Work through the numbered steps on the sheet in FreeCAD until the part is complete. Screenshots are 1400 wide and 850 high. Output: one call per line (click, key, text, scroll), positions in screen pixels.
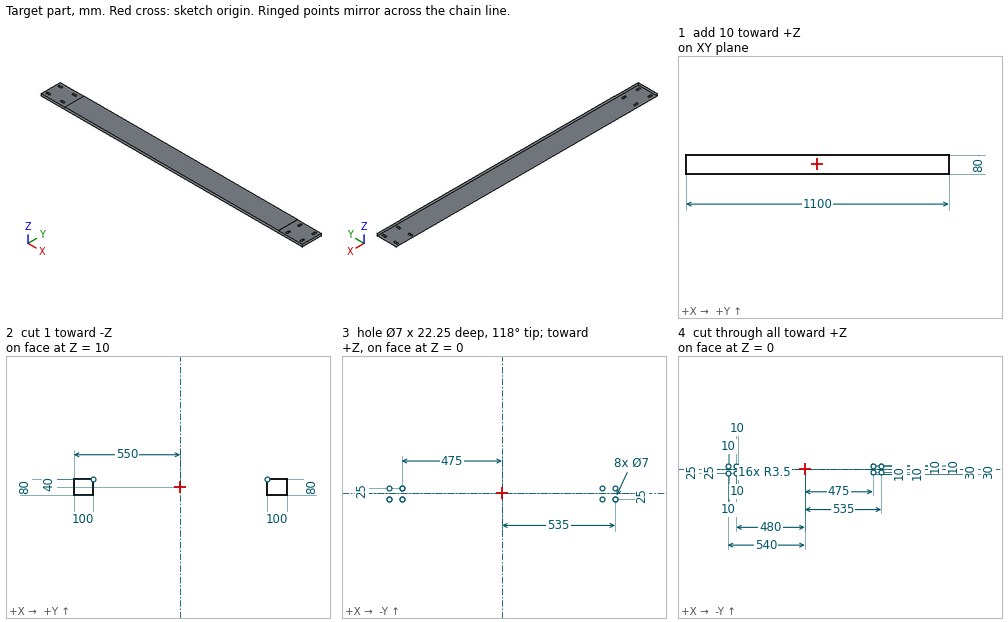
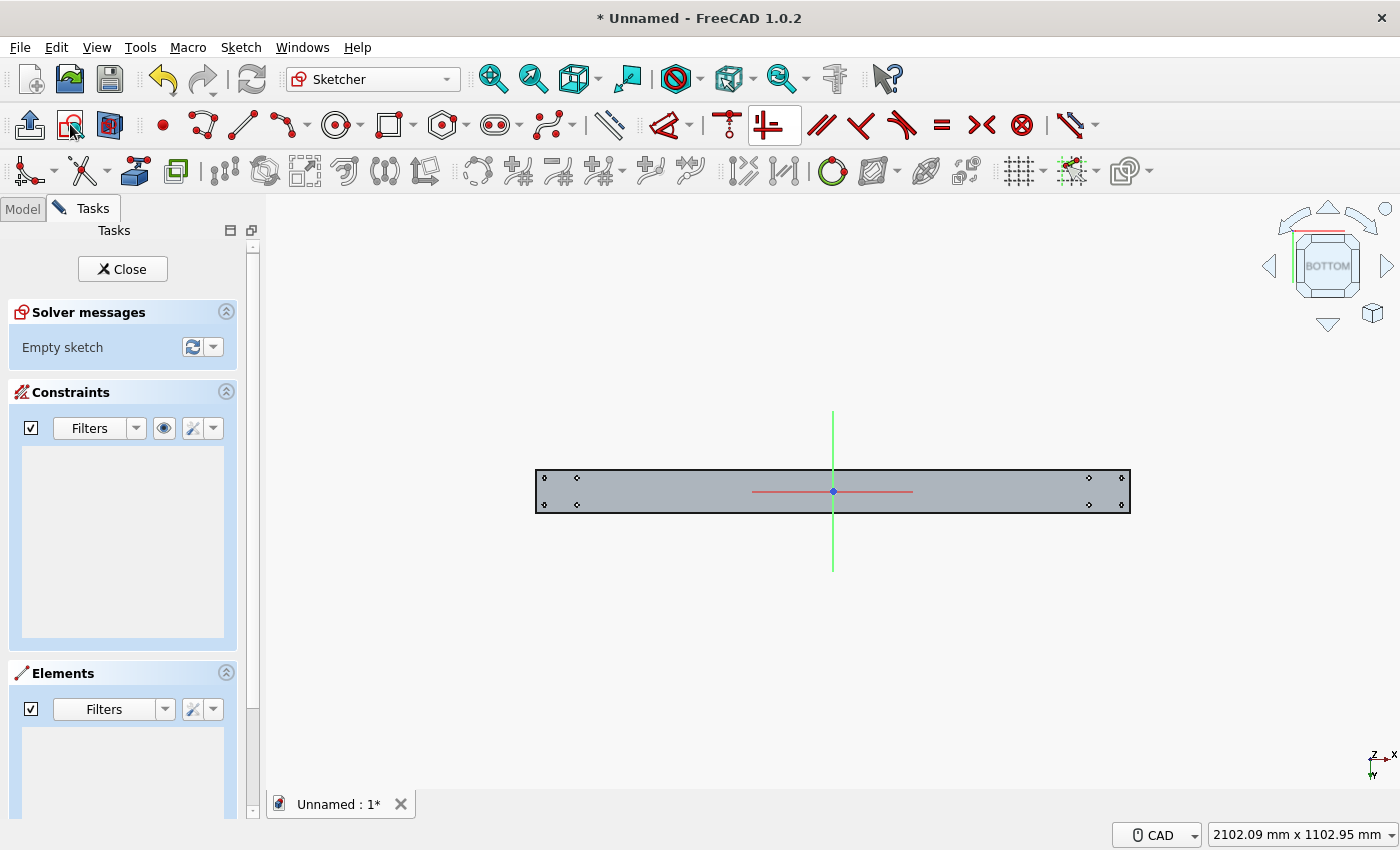
scroll(574, 505, up, 13)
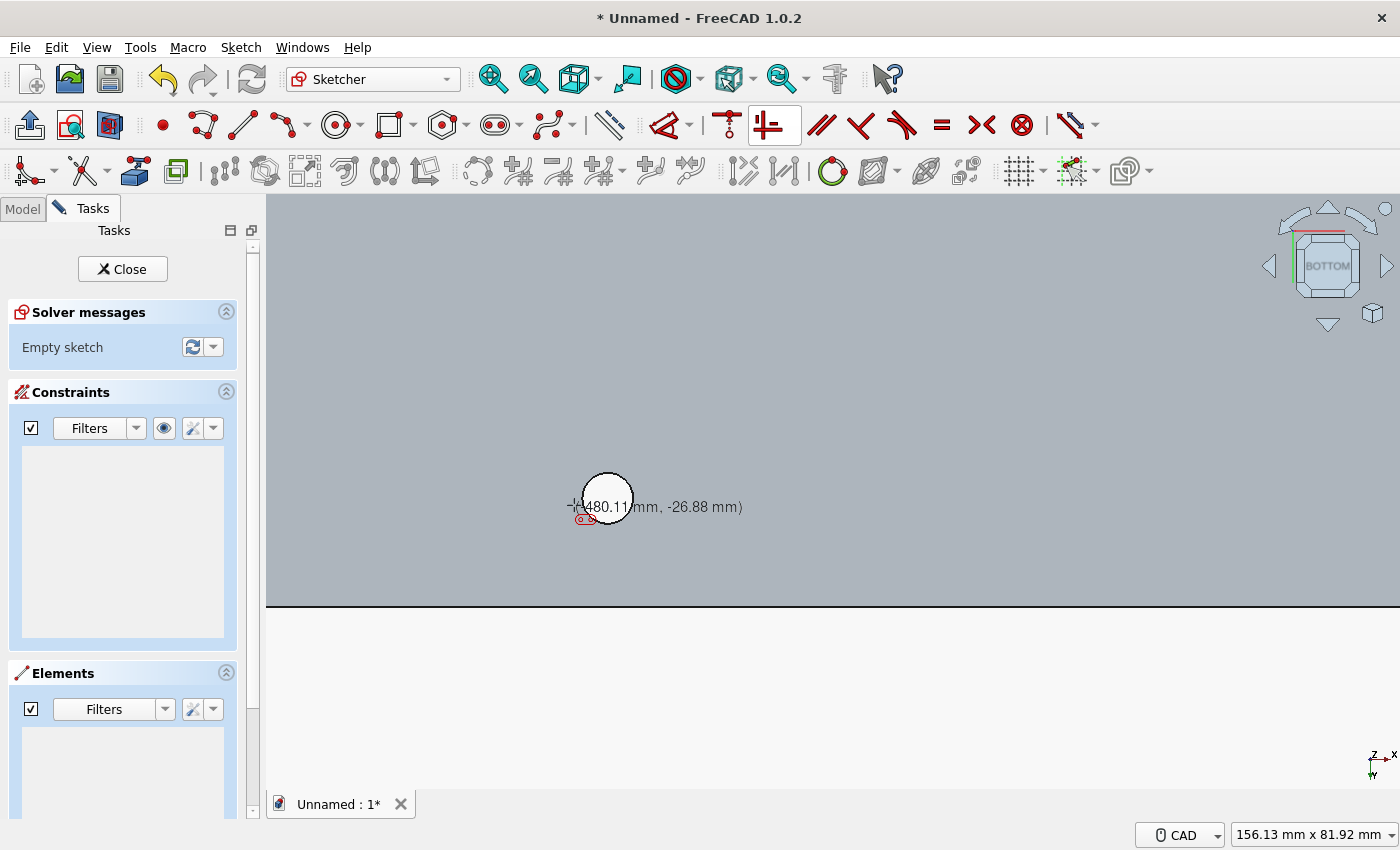
scroll(438, 509, down, 12)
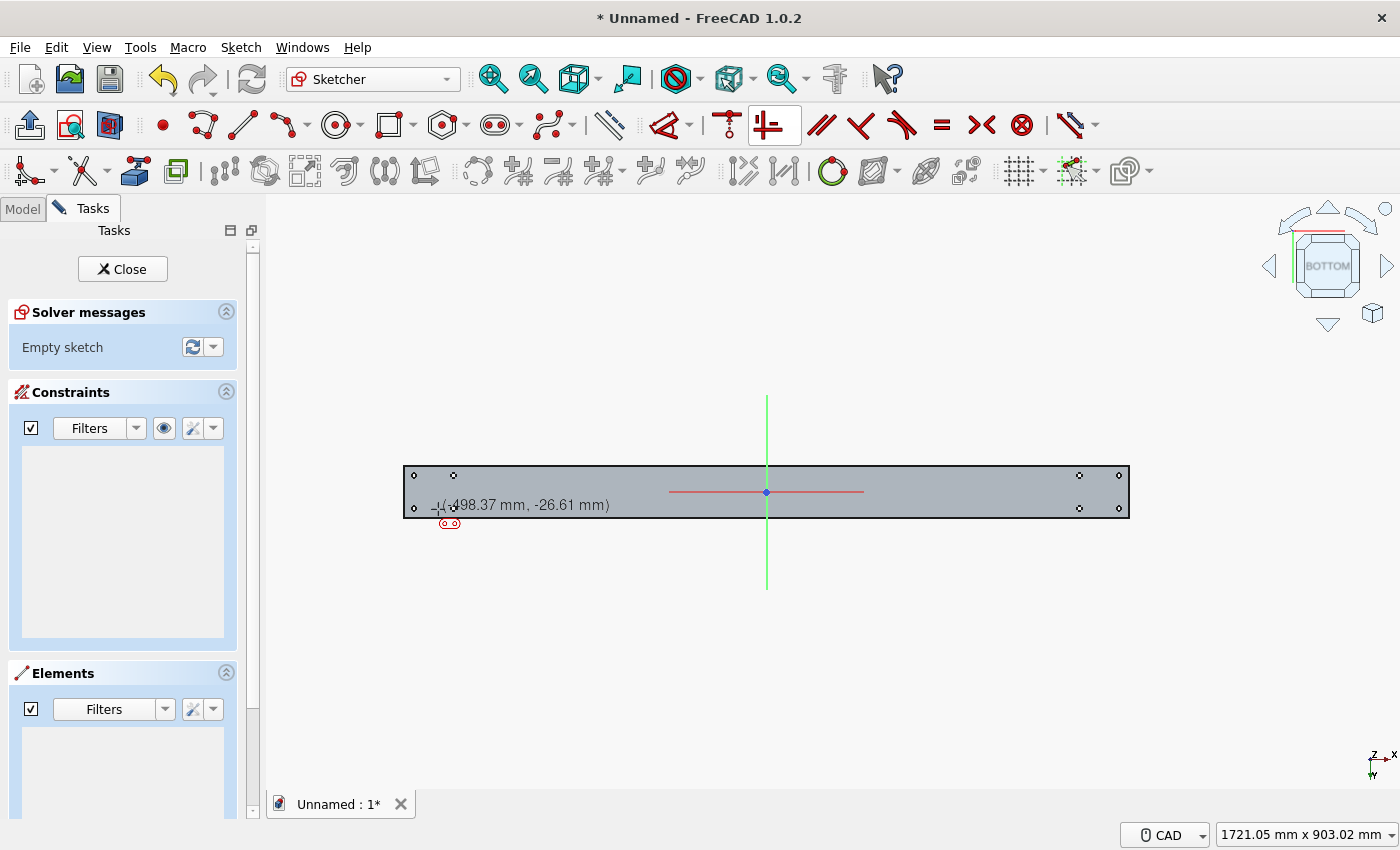
click(450, 509)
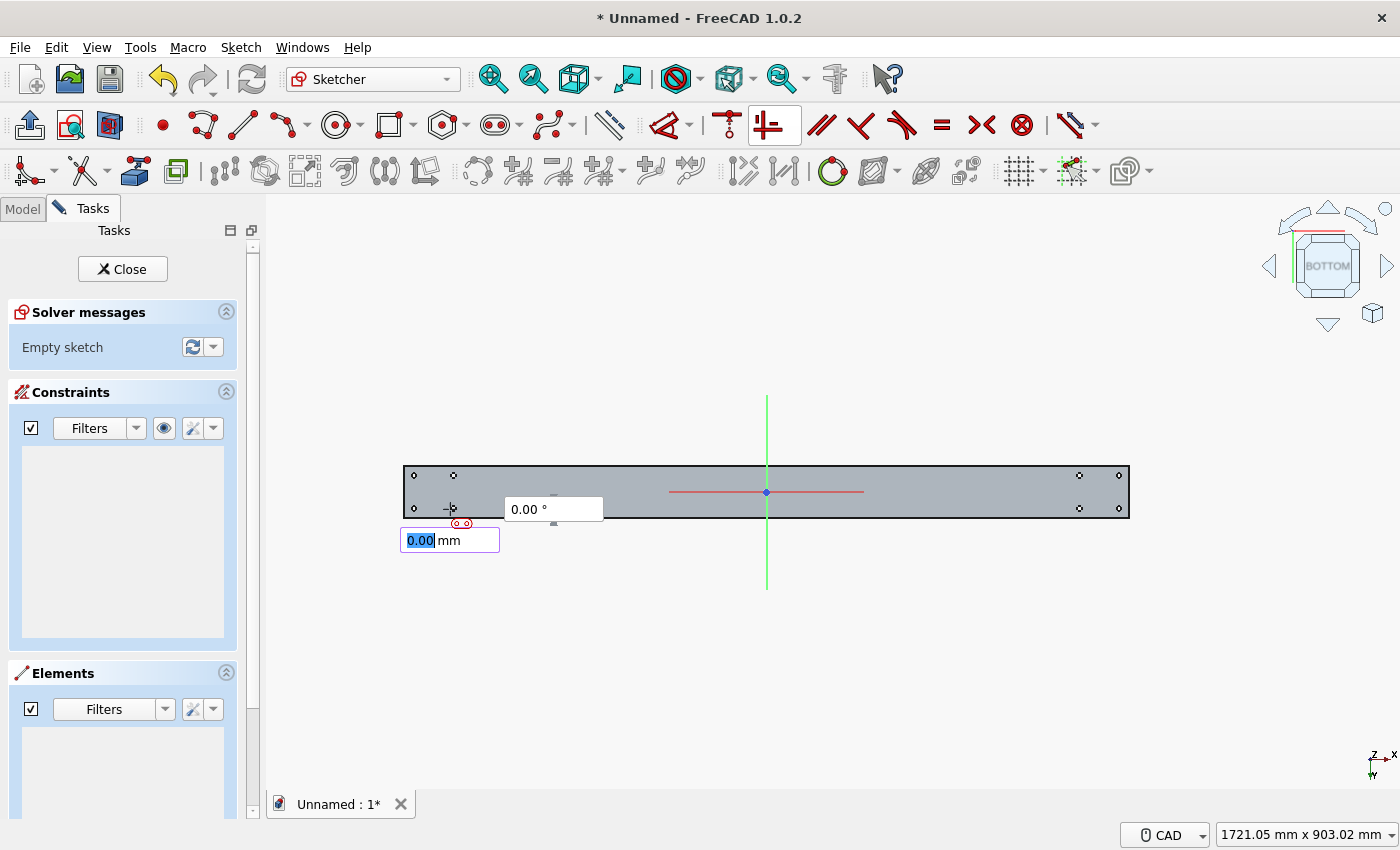
scroll(457, 509, up, 5)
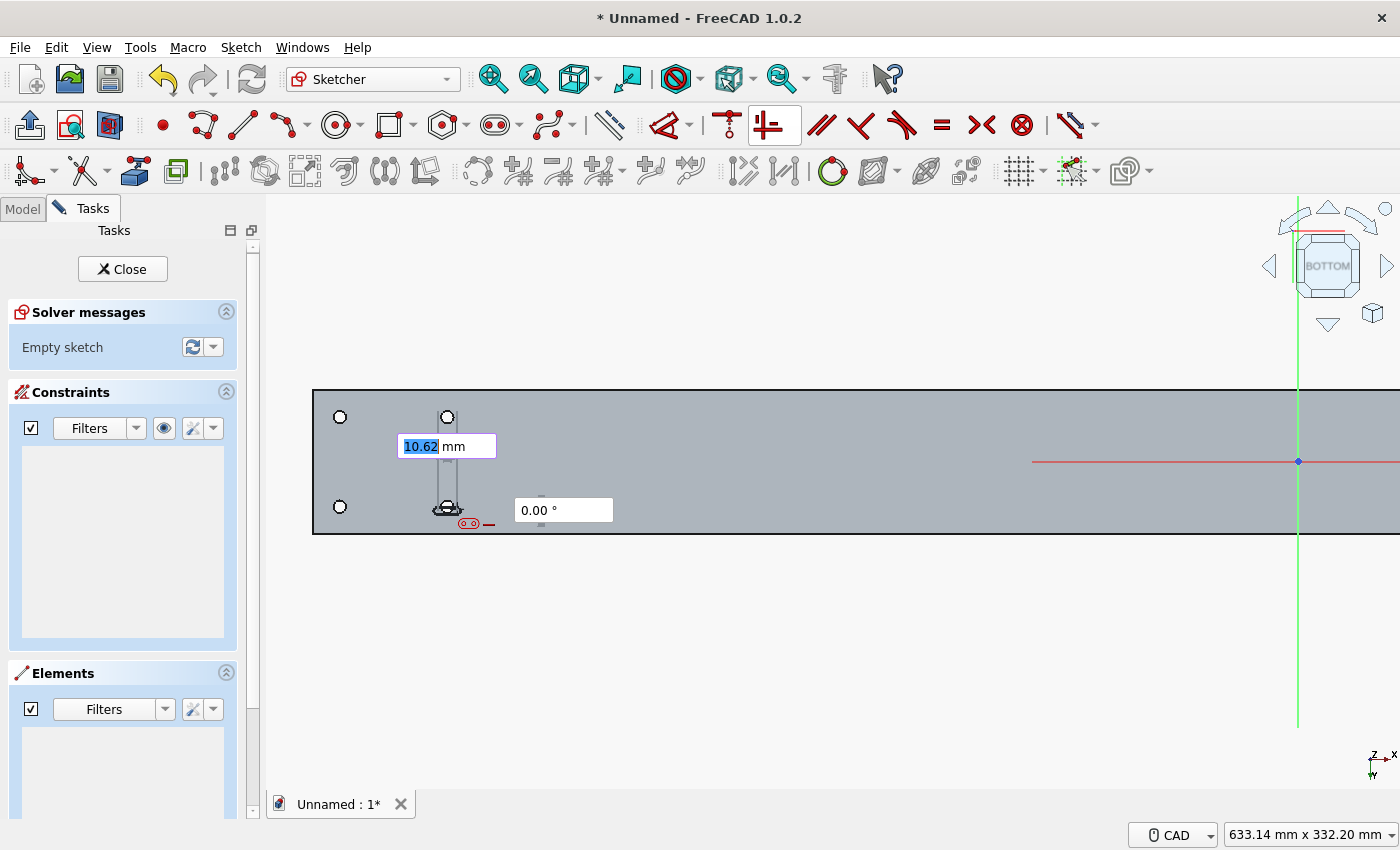
click(456, 508)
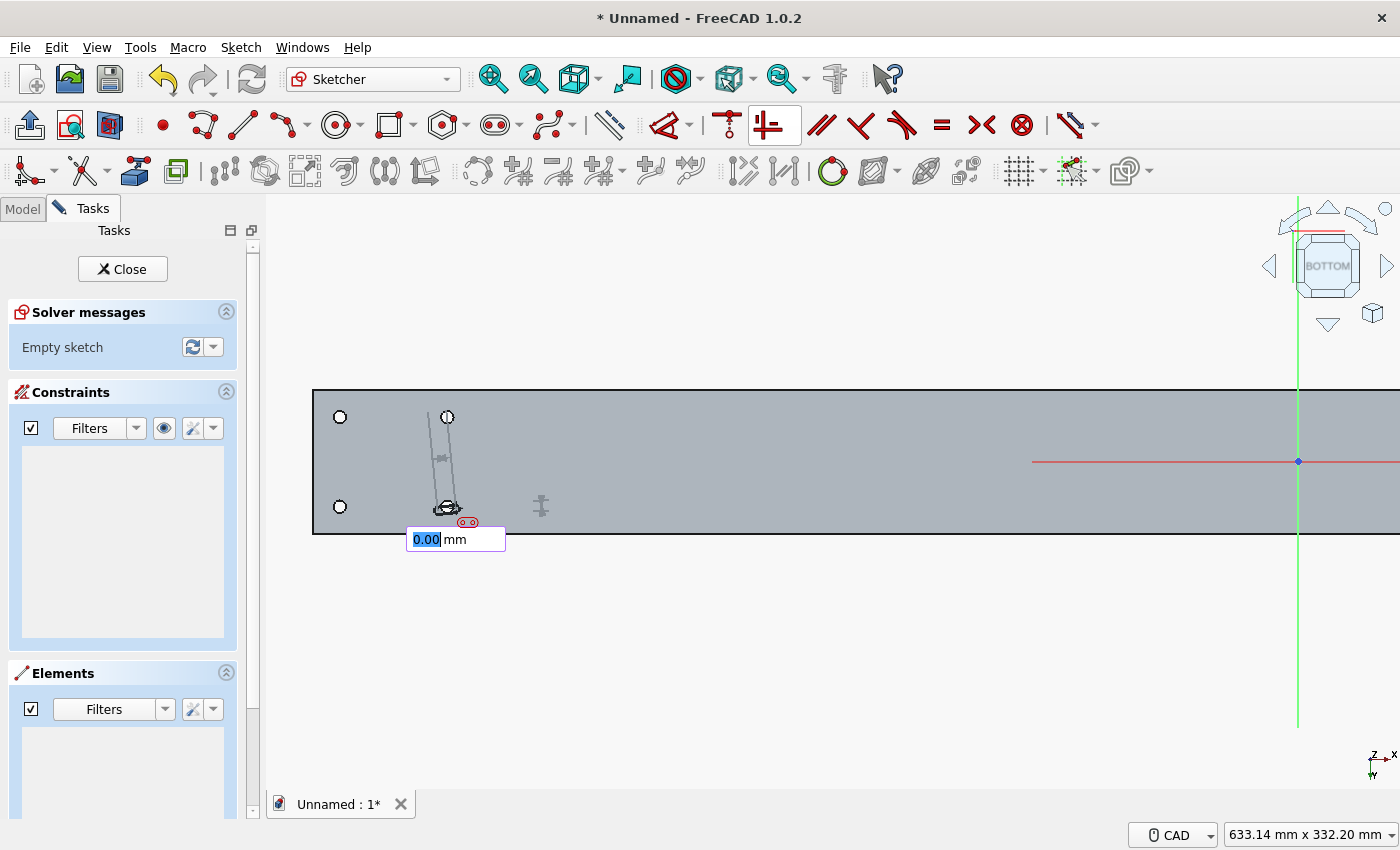
scroll(447, 513, up, 5)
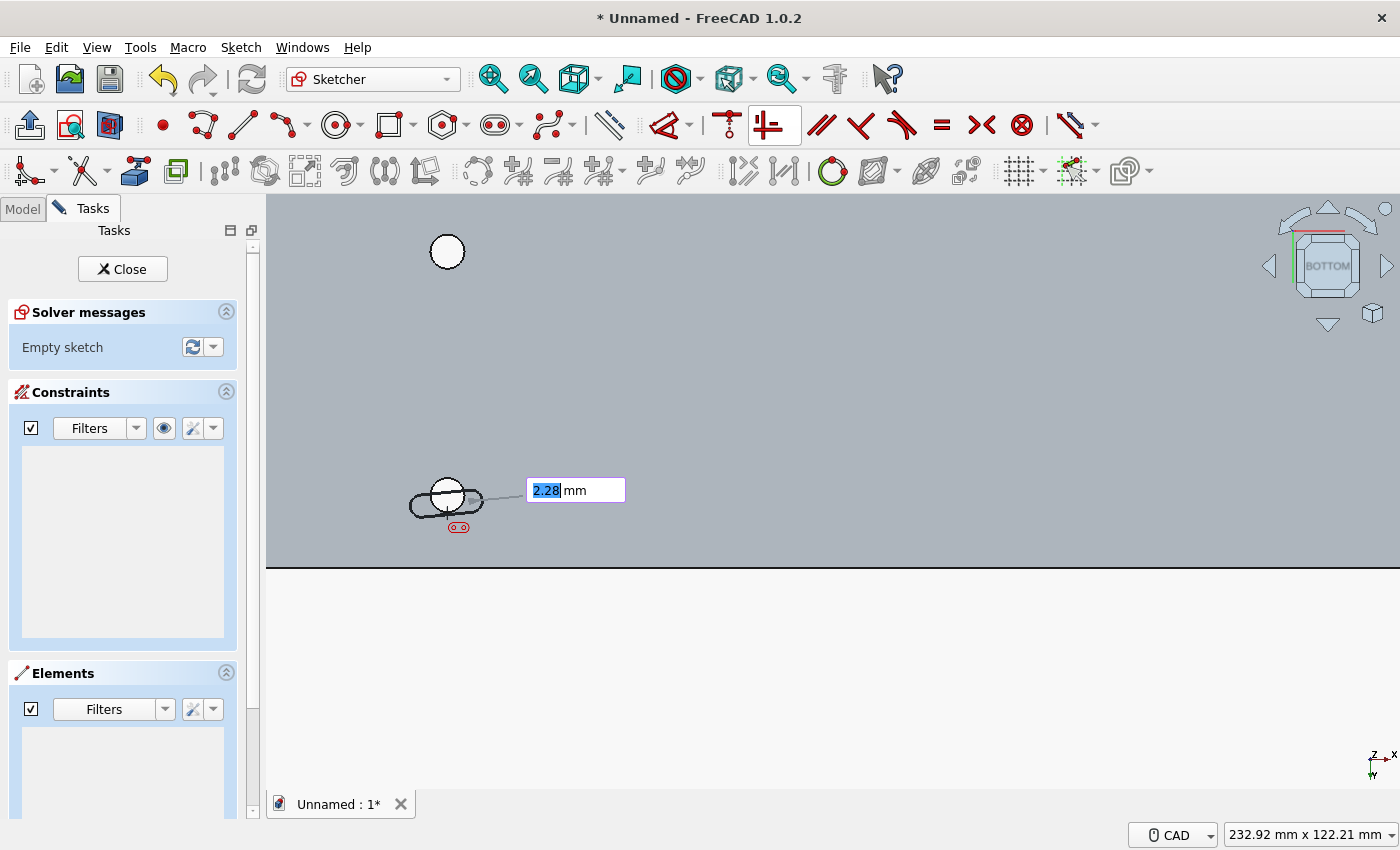
click(448, 512)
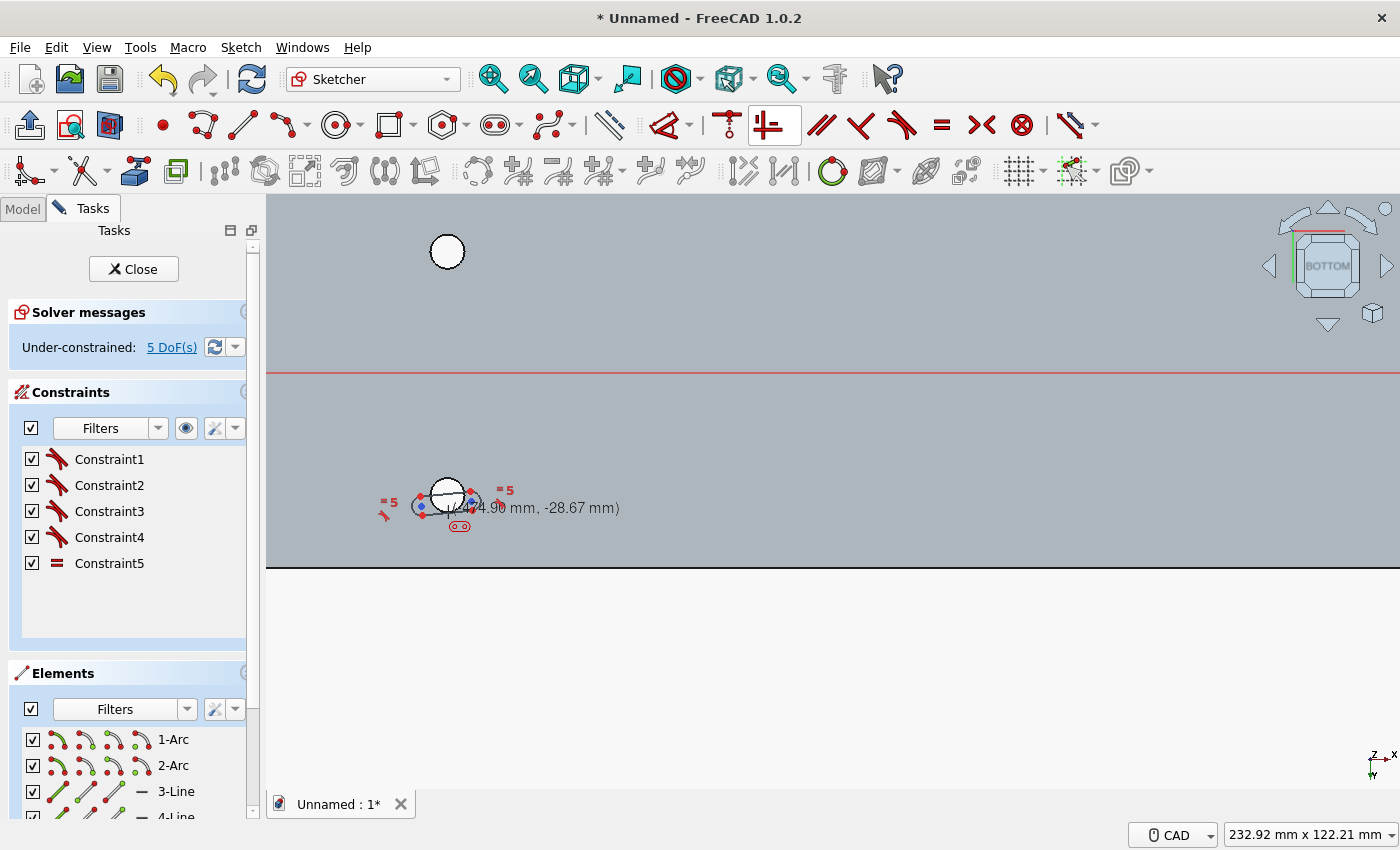
scroll(454, 510, down, 10)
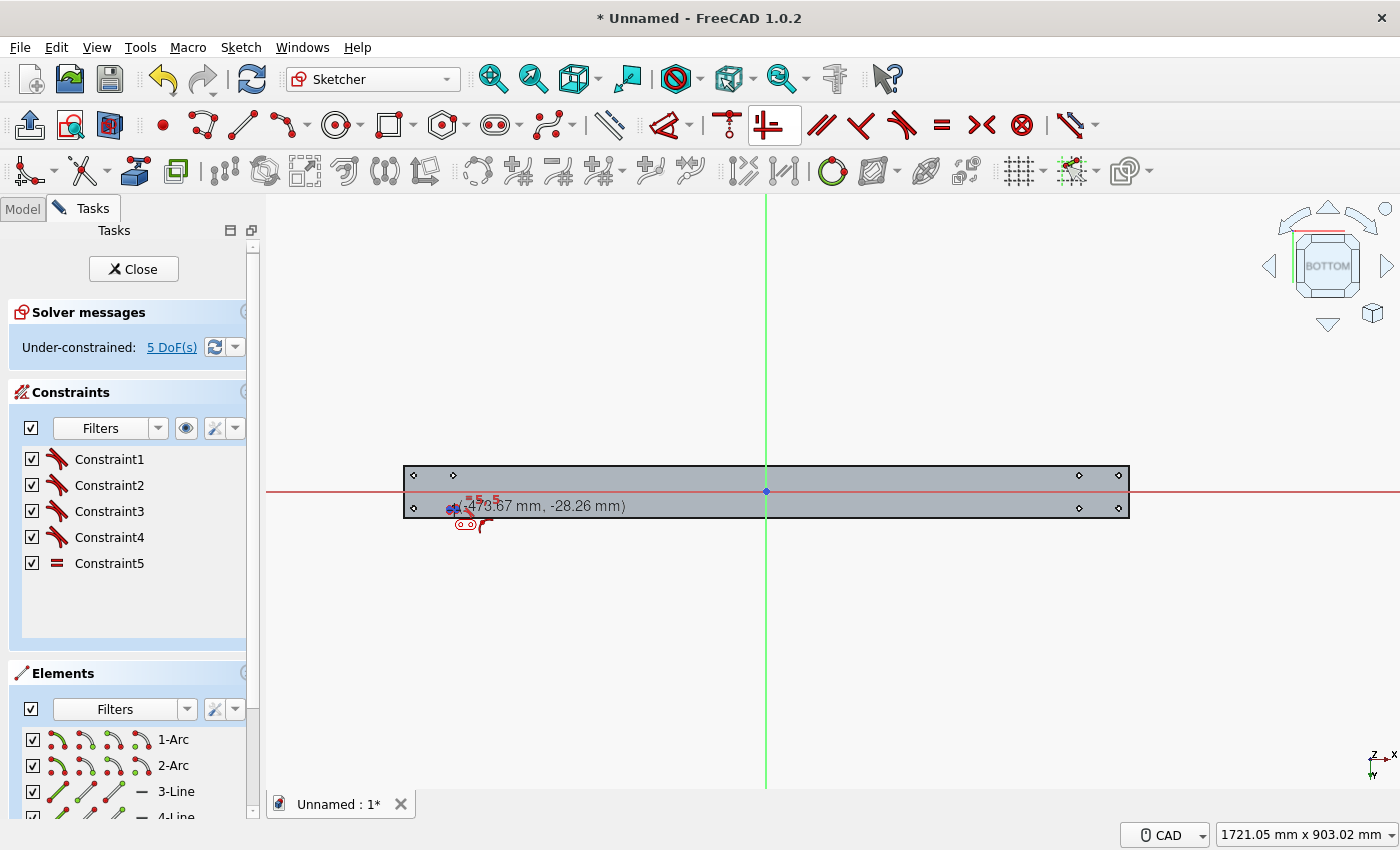
scroll(410, 508, up, 12)